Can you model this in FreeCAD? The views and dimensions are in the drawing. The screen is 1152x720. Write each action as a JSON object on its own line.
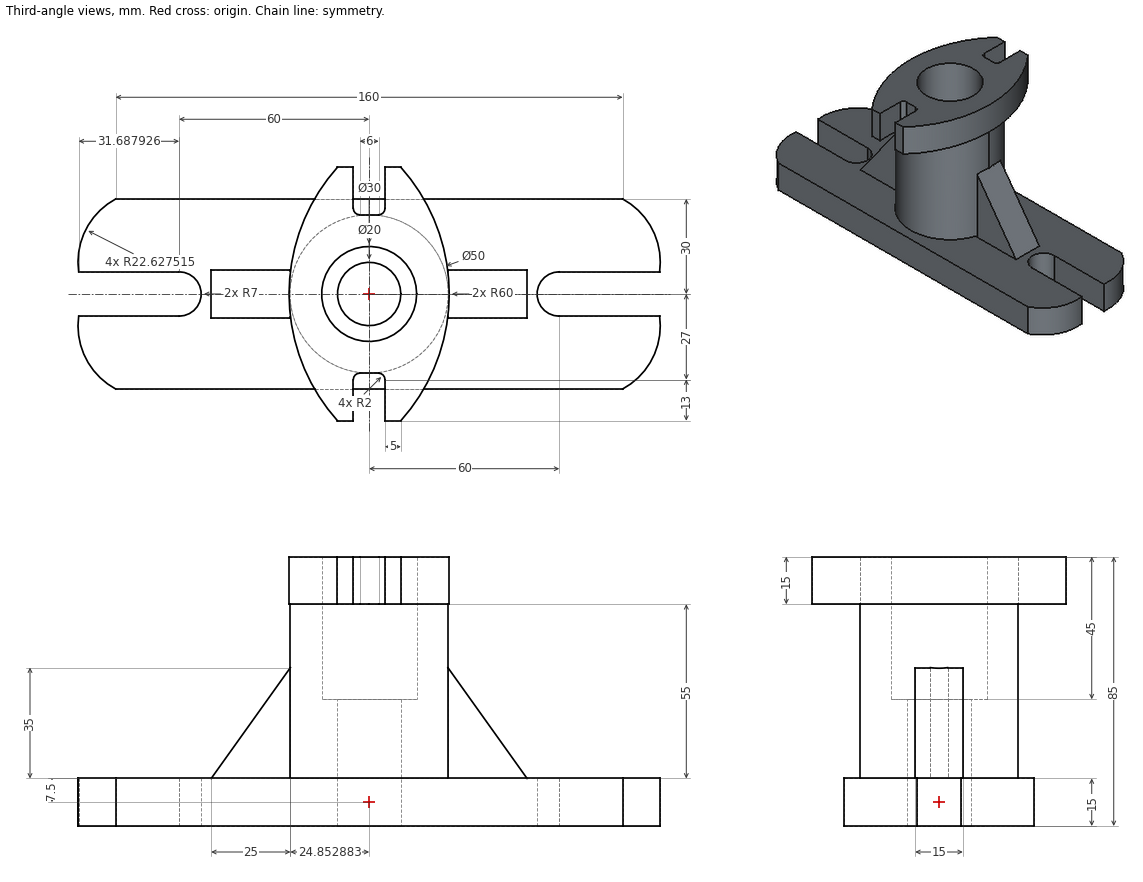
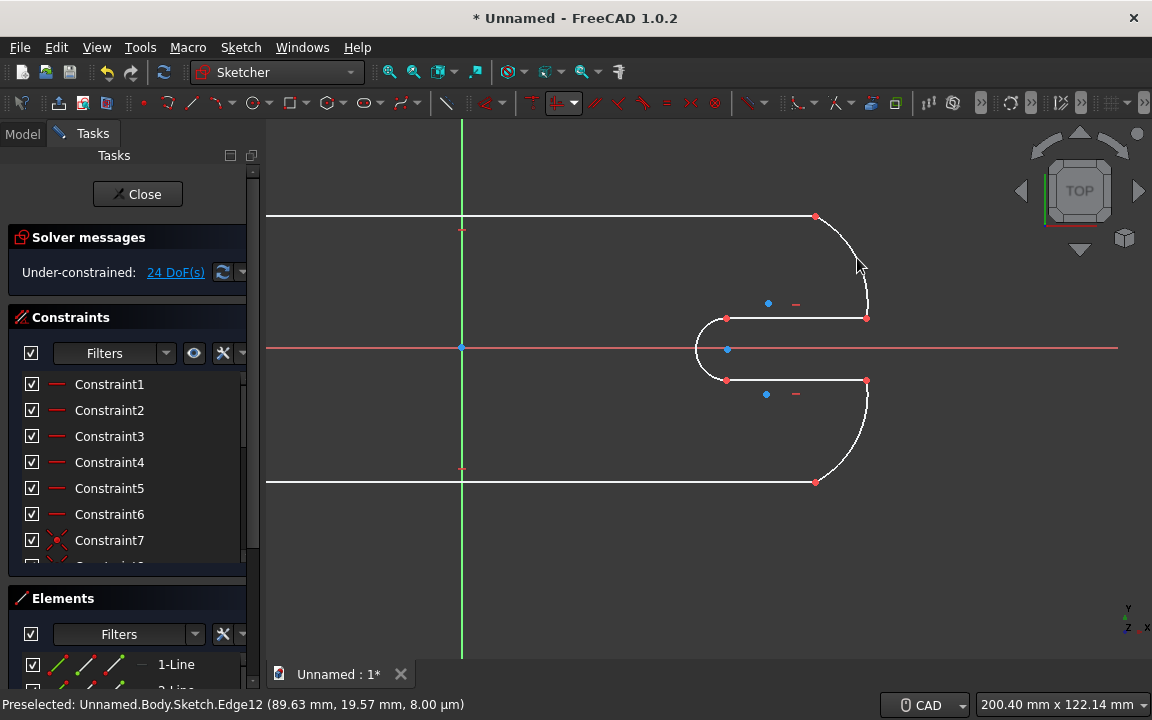
{"action": "scroll", "coordinate": [858, 439], "scroll_direction": "down", "scroll_amount": 3}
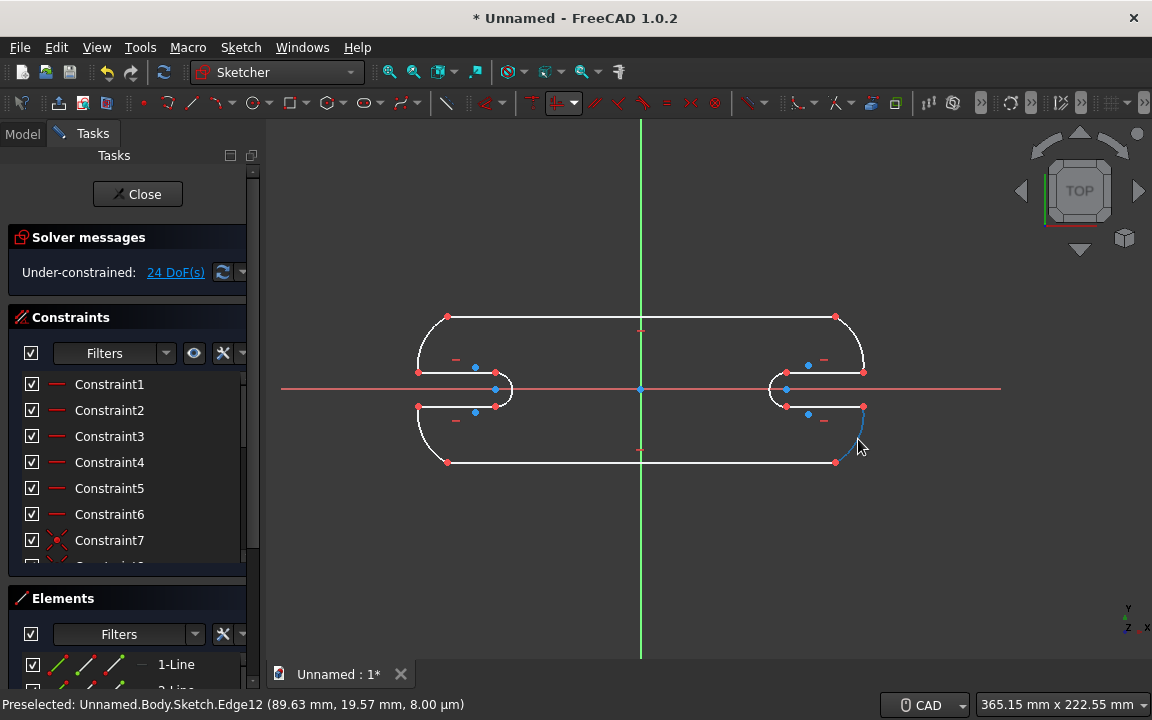
{"action": "left_click", "coordinate": [441, 373]}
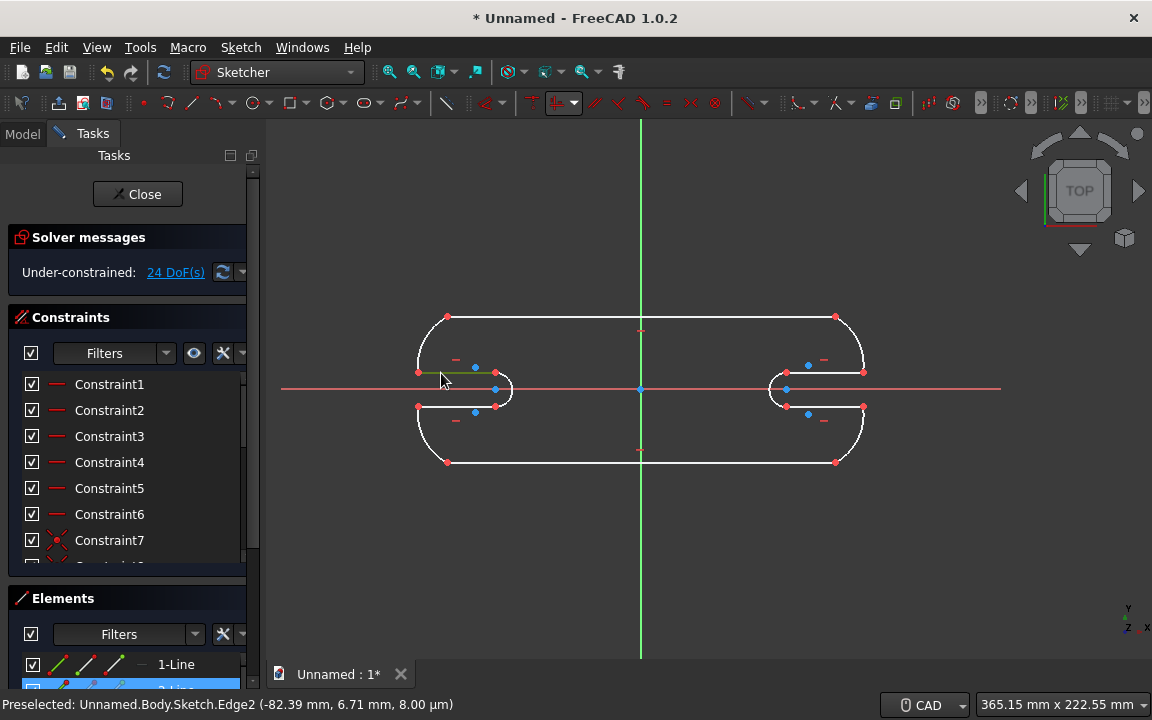
{"action": "scroll", "coordinate": [509, 400], "scroll_direction": "up", "scroll_amount": 2}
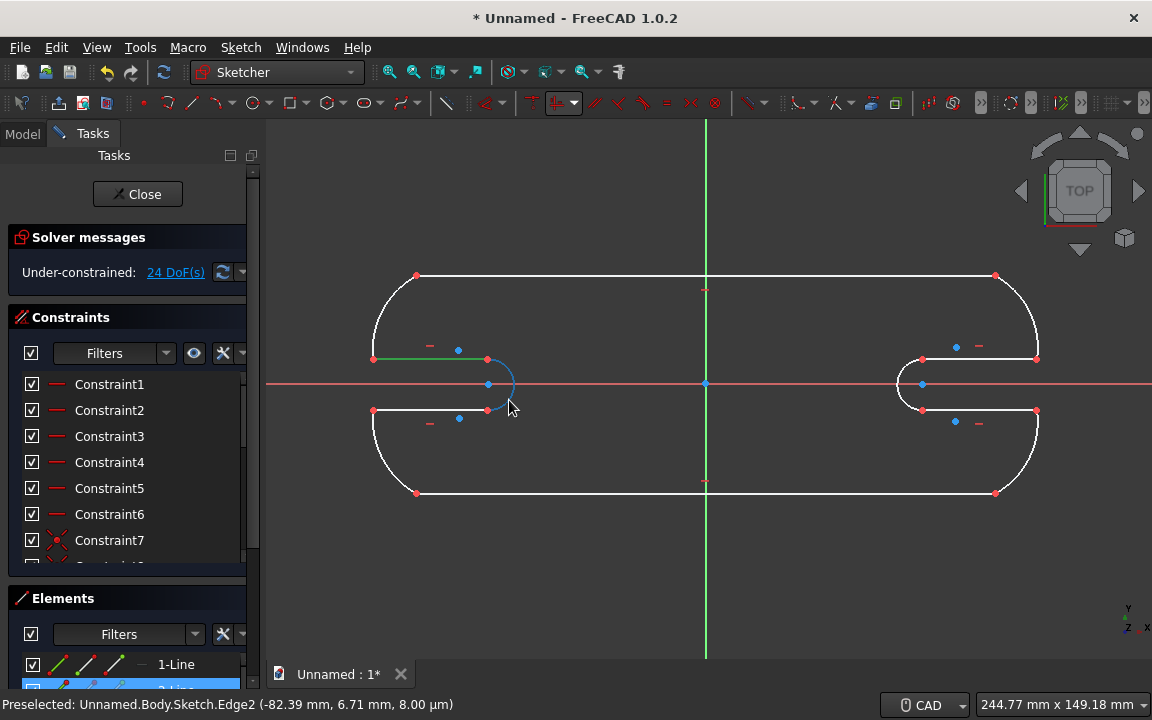
{"action": "left_click", "coordinate": [509, 400]}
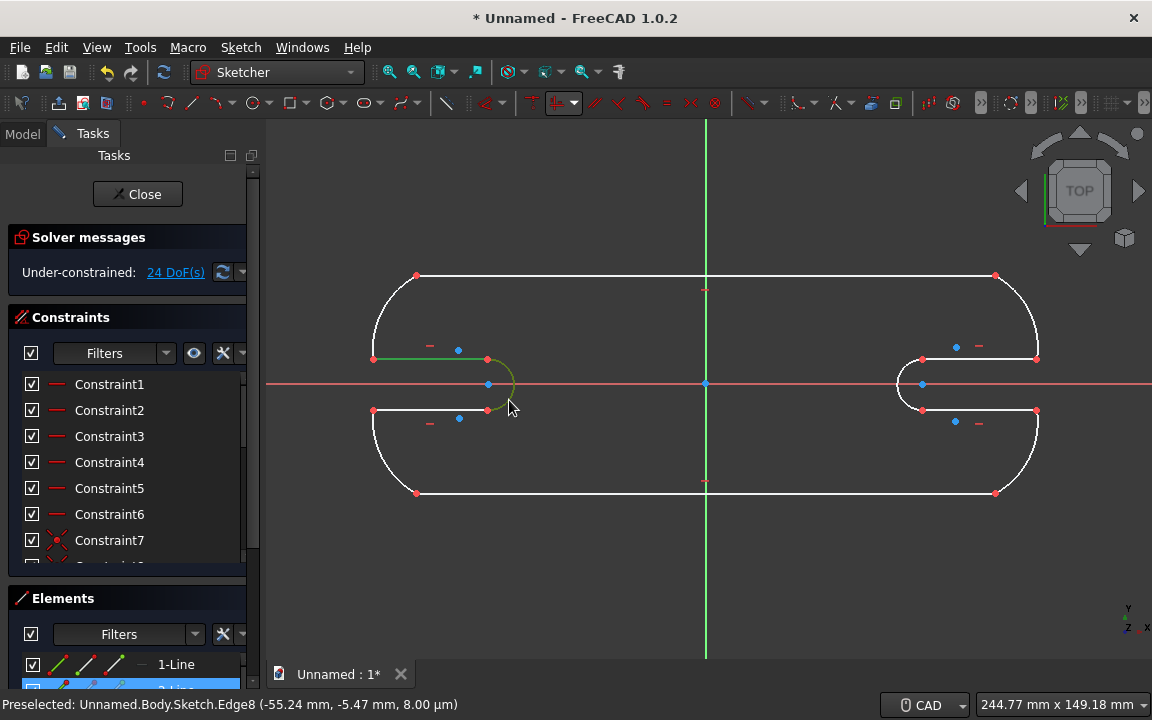
{"action": "key", "text": "t"}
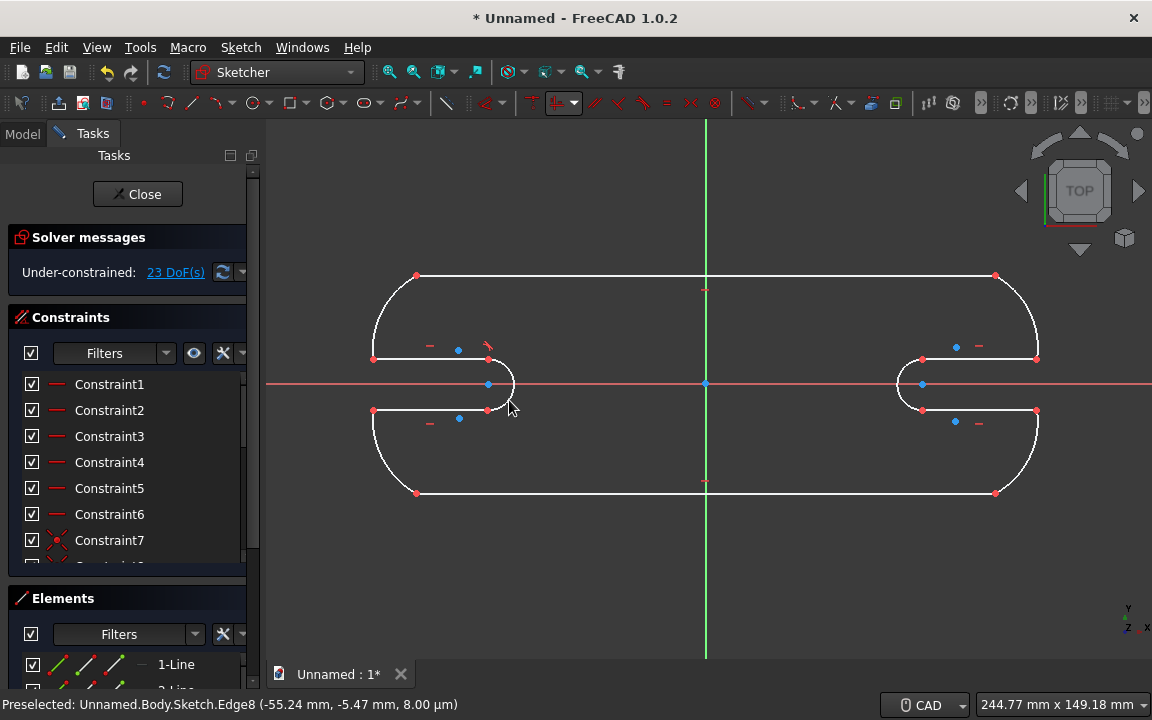
{"action": "left_click", "coordinate": [454, 410]}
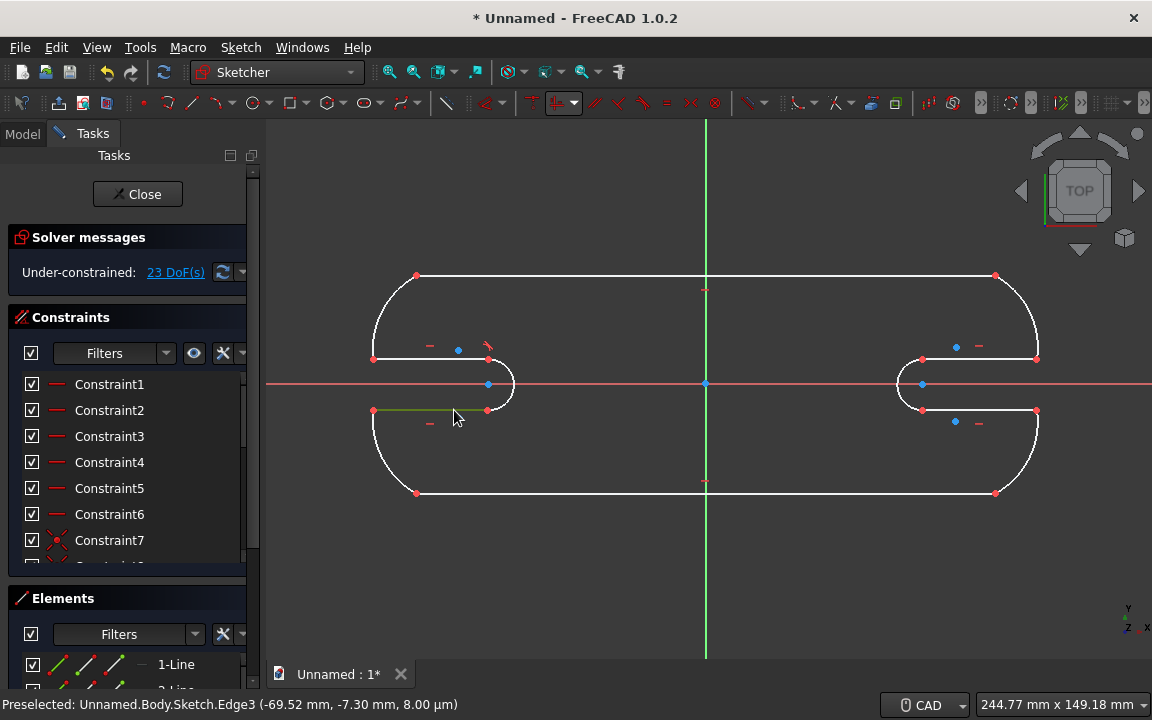
{"action": "left_click", "coordinate": [509, 400]}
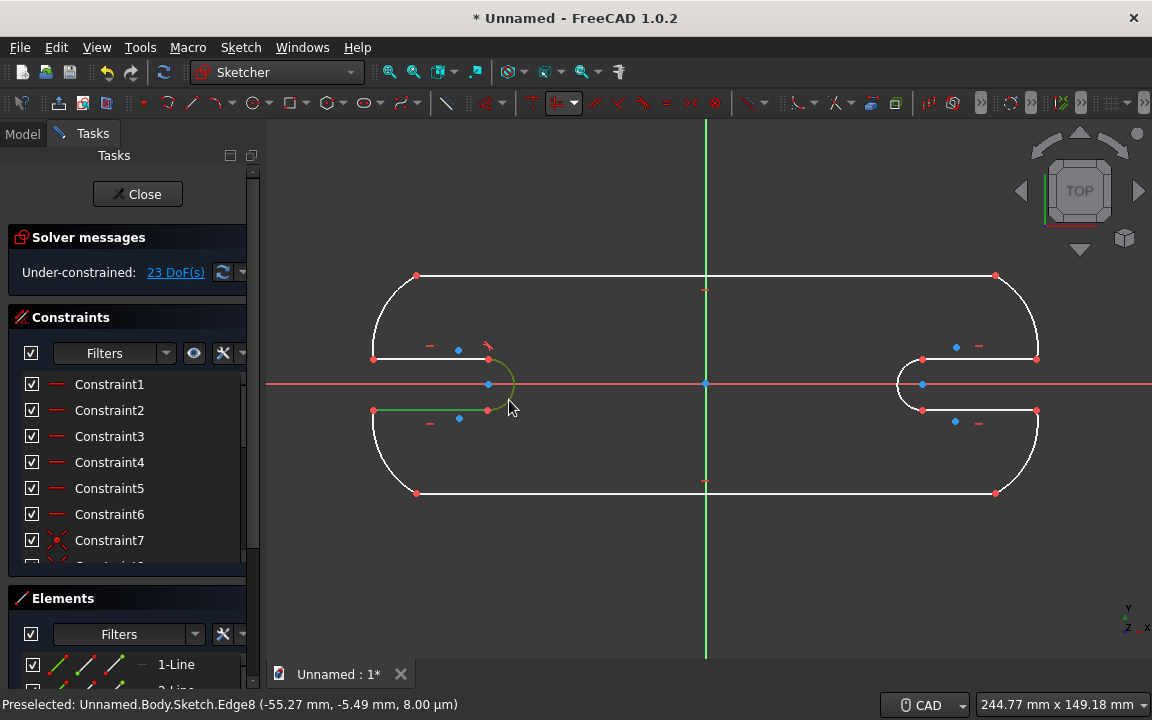
{"action": "key", "text": "t"}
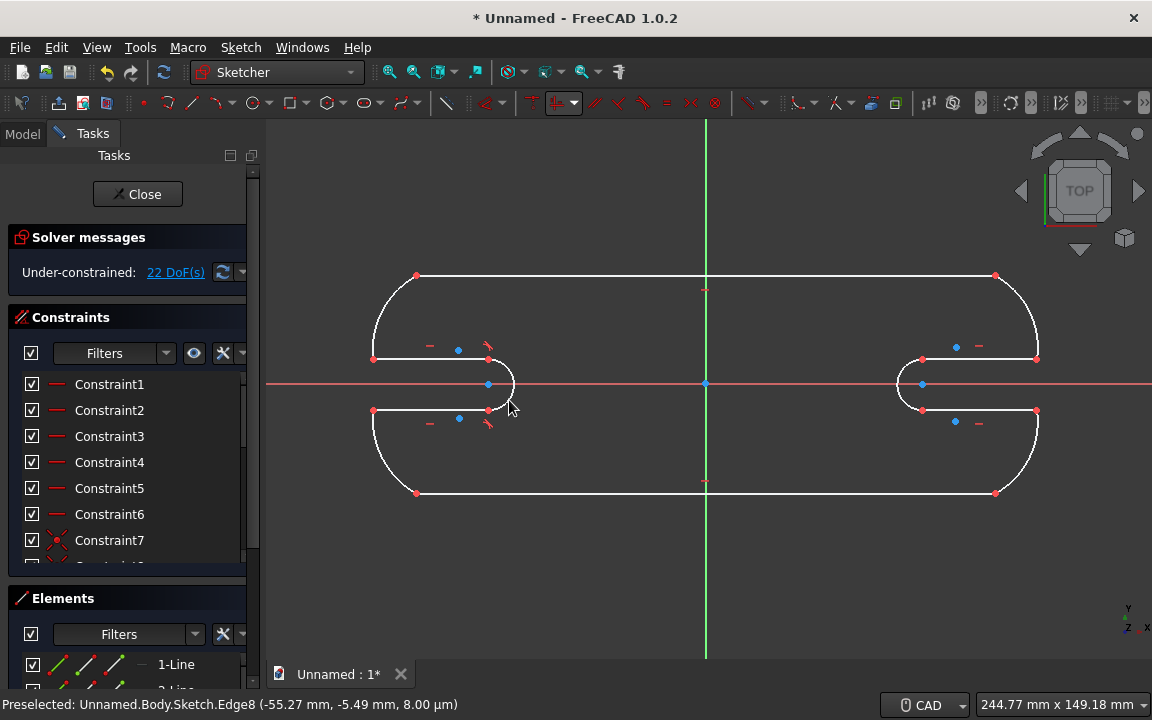
{"action": "left_click", "coordinate": [957, 410]}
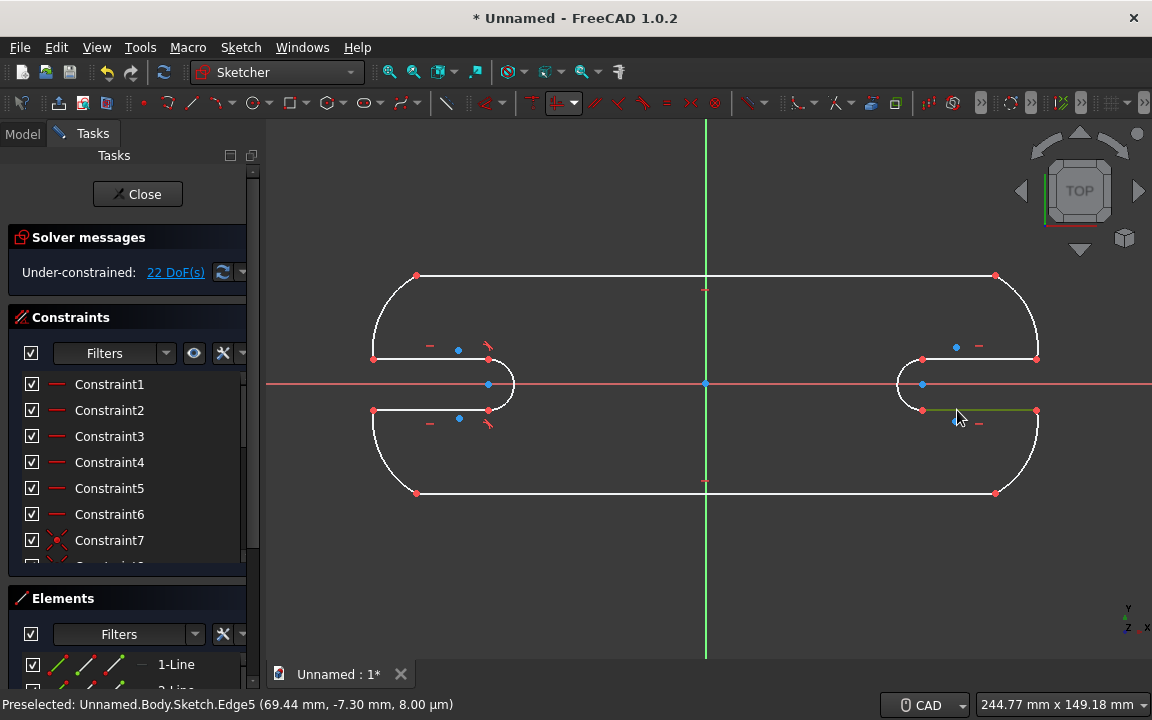
{"action": "left_click", "coordinate": [902, 370]}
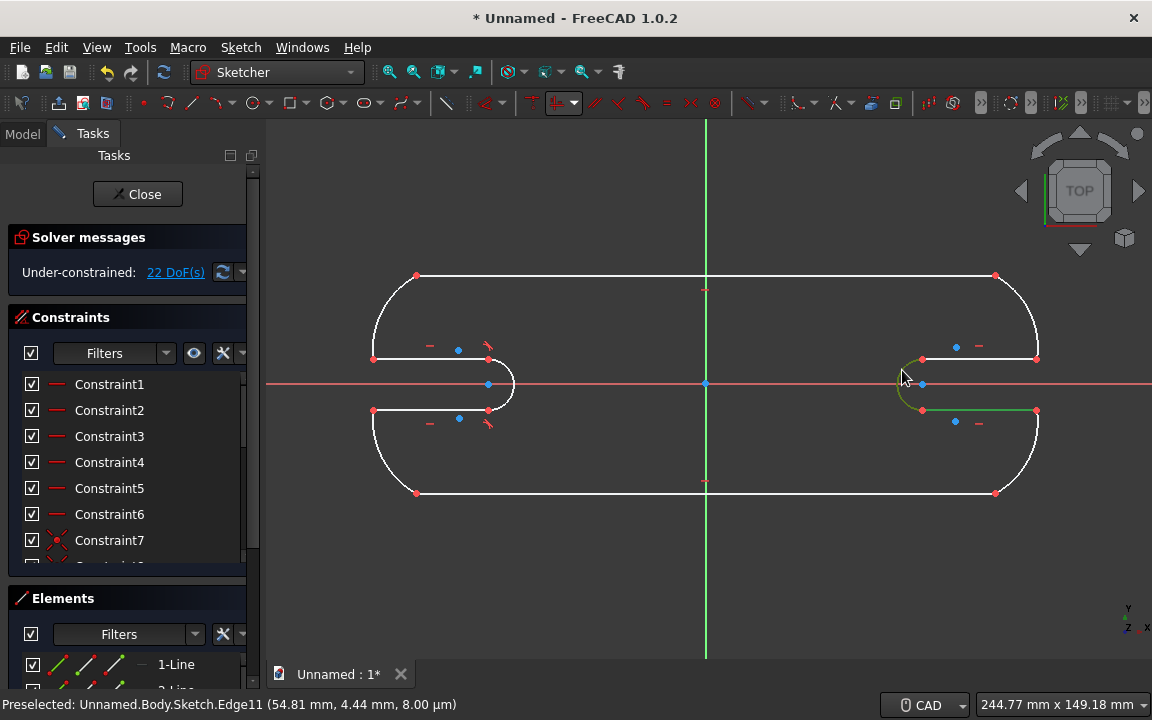
{"action": "key", "text": "t"}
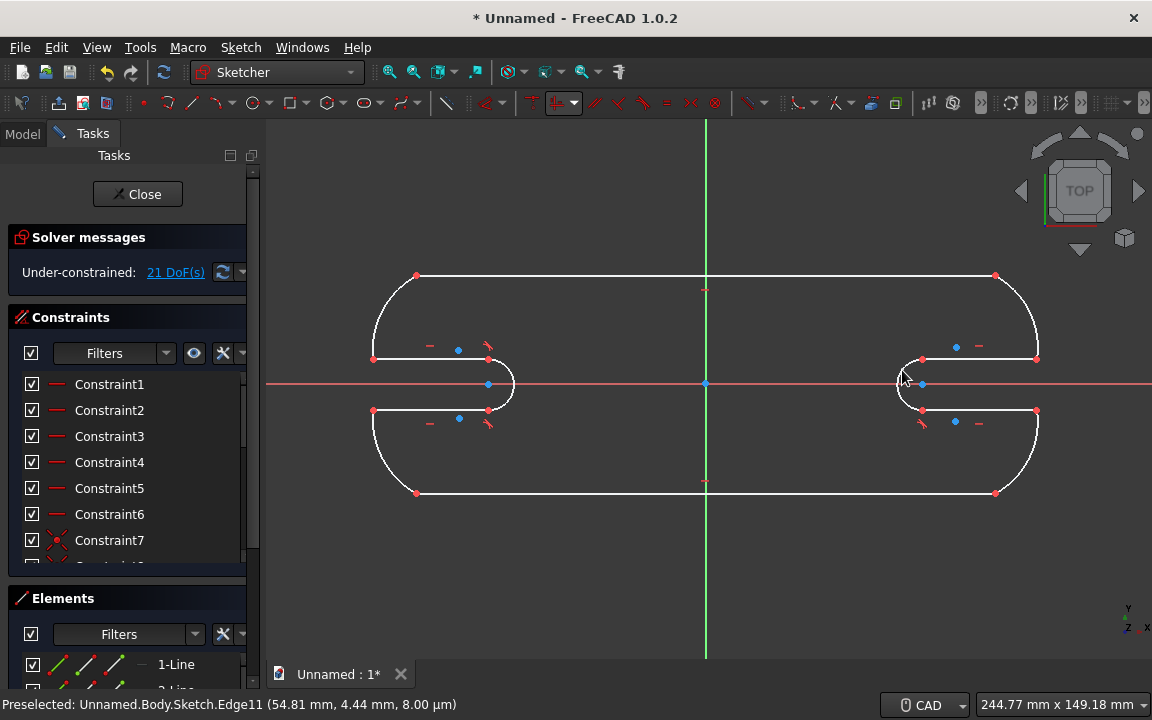
{"action": "left_click", "coordinate": [957, 359]}